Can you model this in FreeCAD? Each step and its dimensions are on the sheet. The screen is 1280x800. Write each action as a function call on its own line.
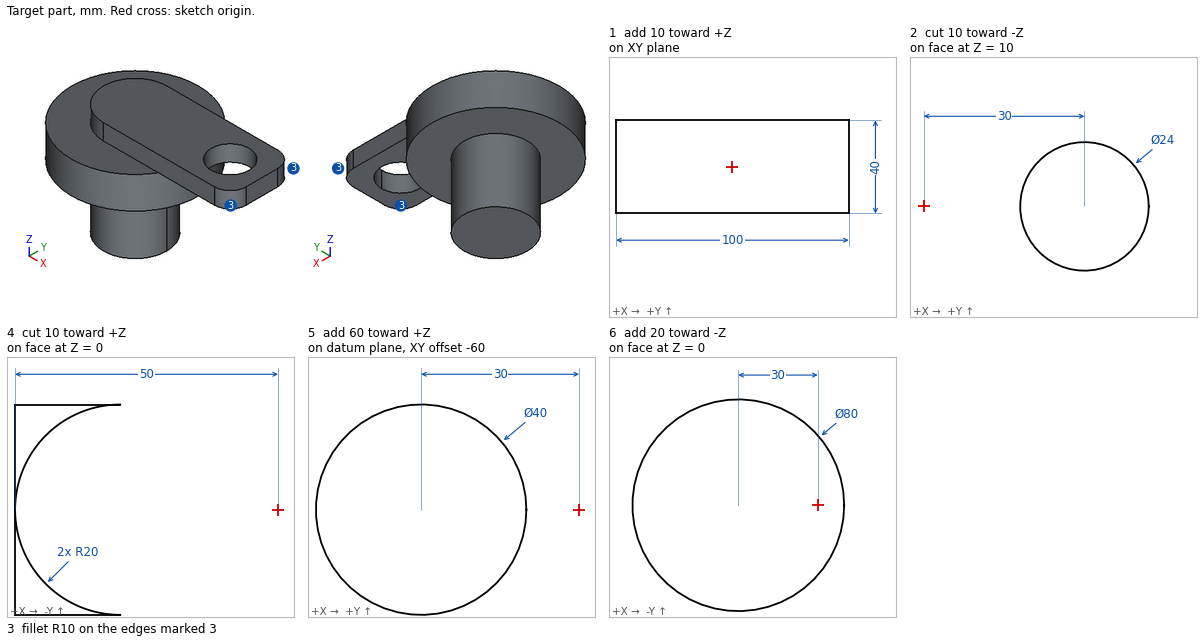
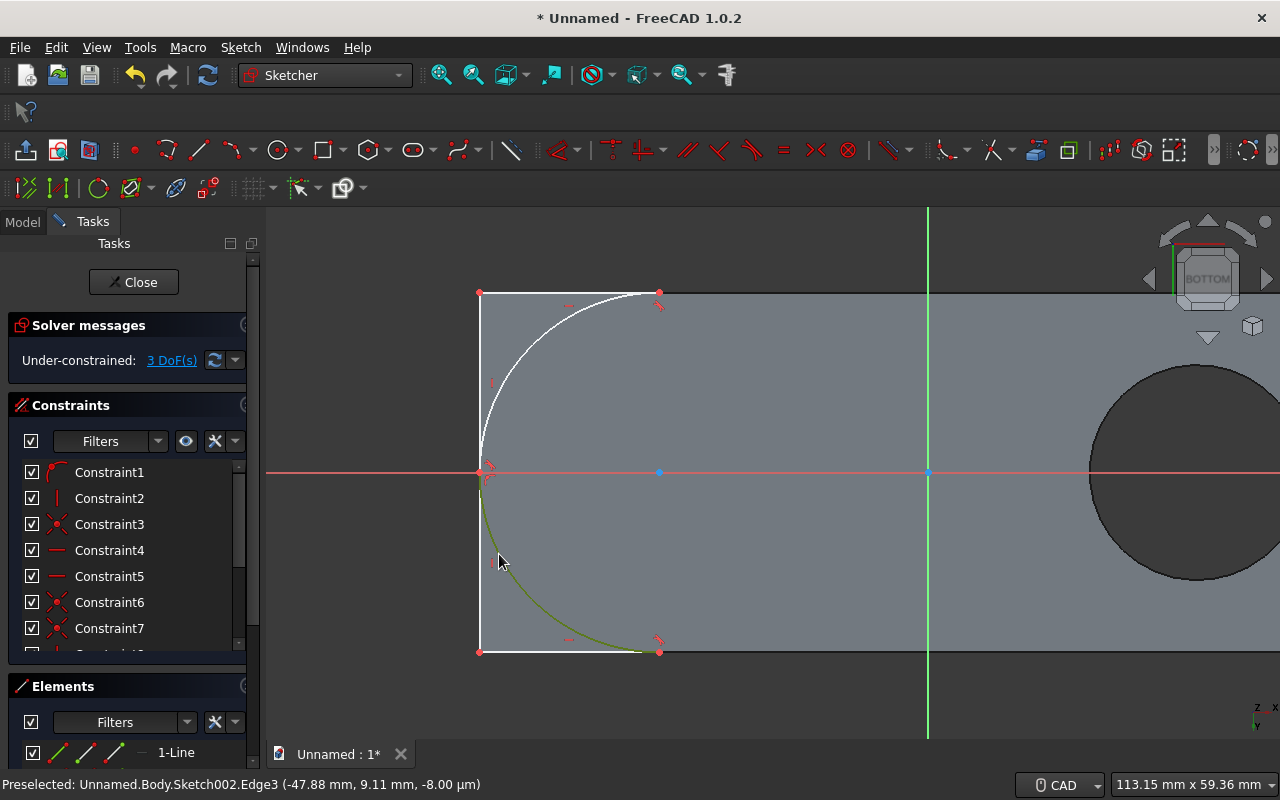
click(578, 312)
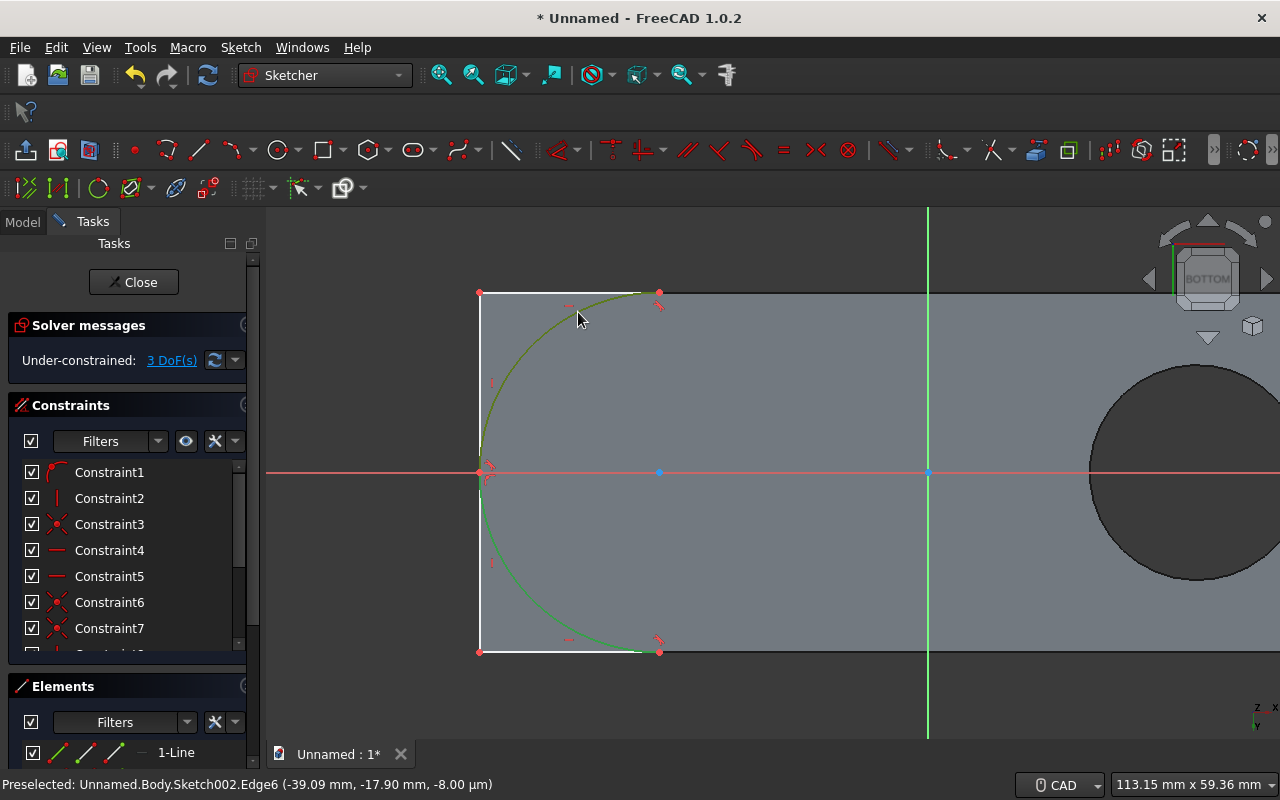
click(784, 150)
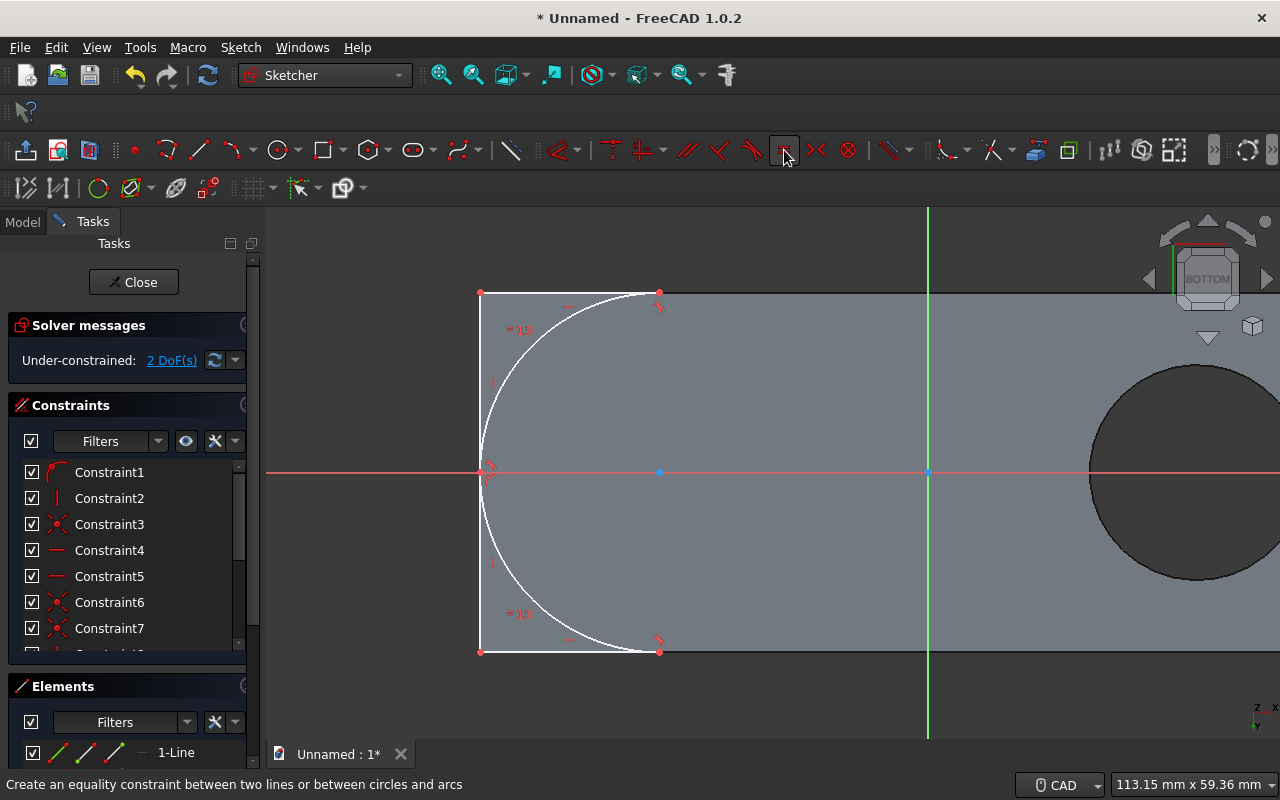
click(500, 554)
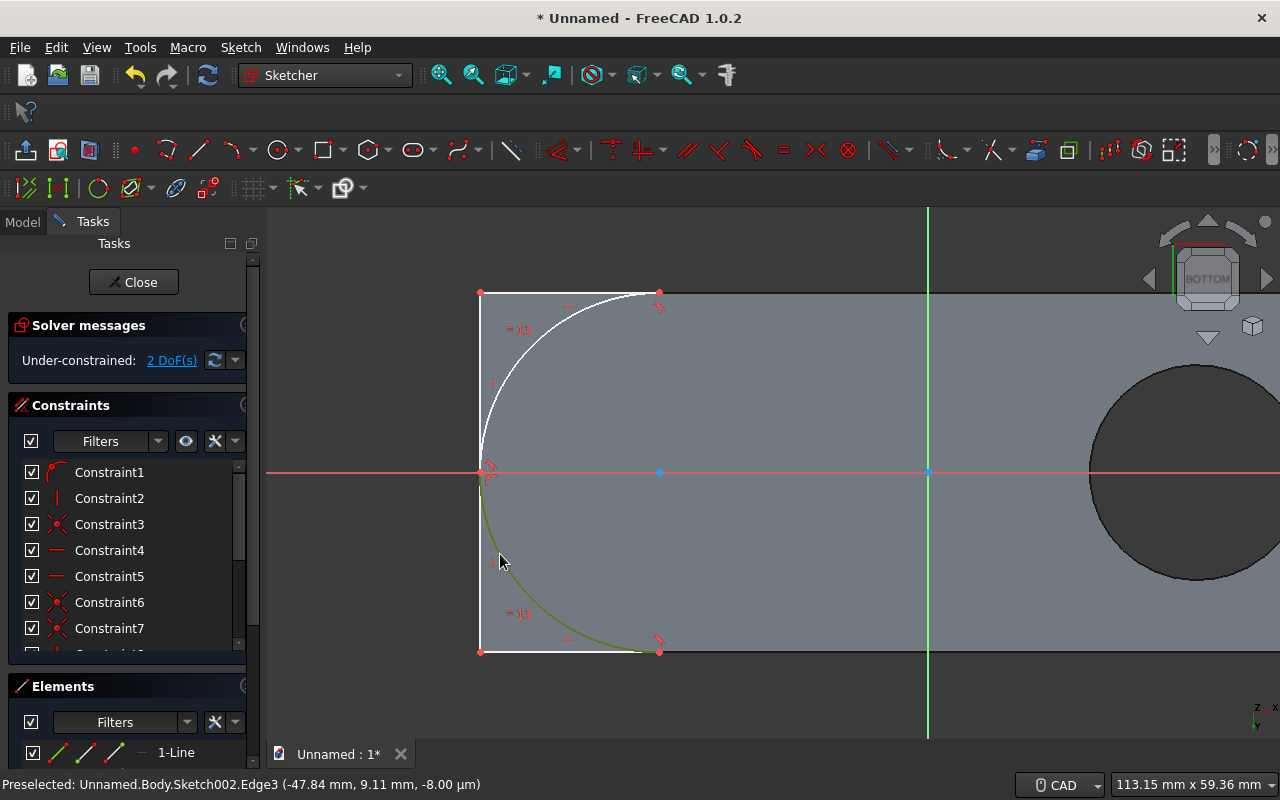
click(580, 150)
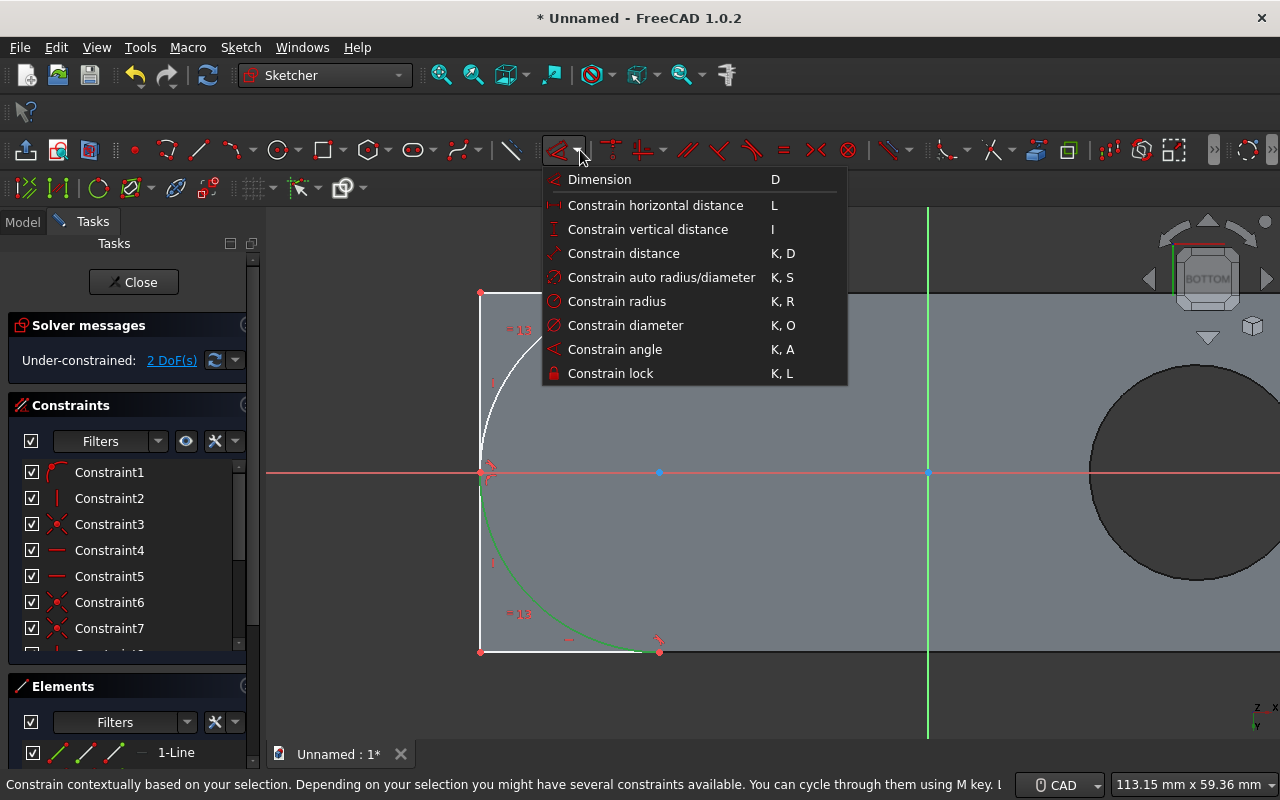
click(695, 301)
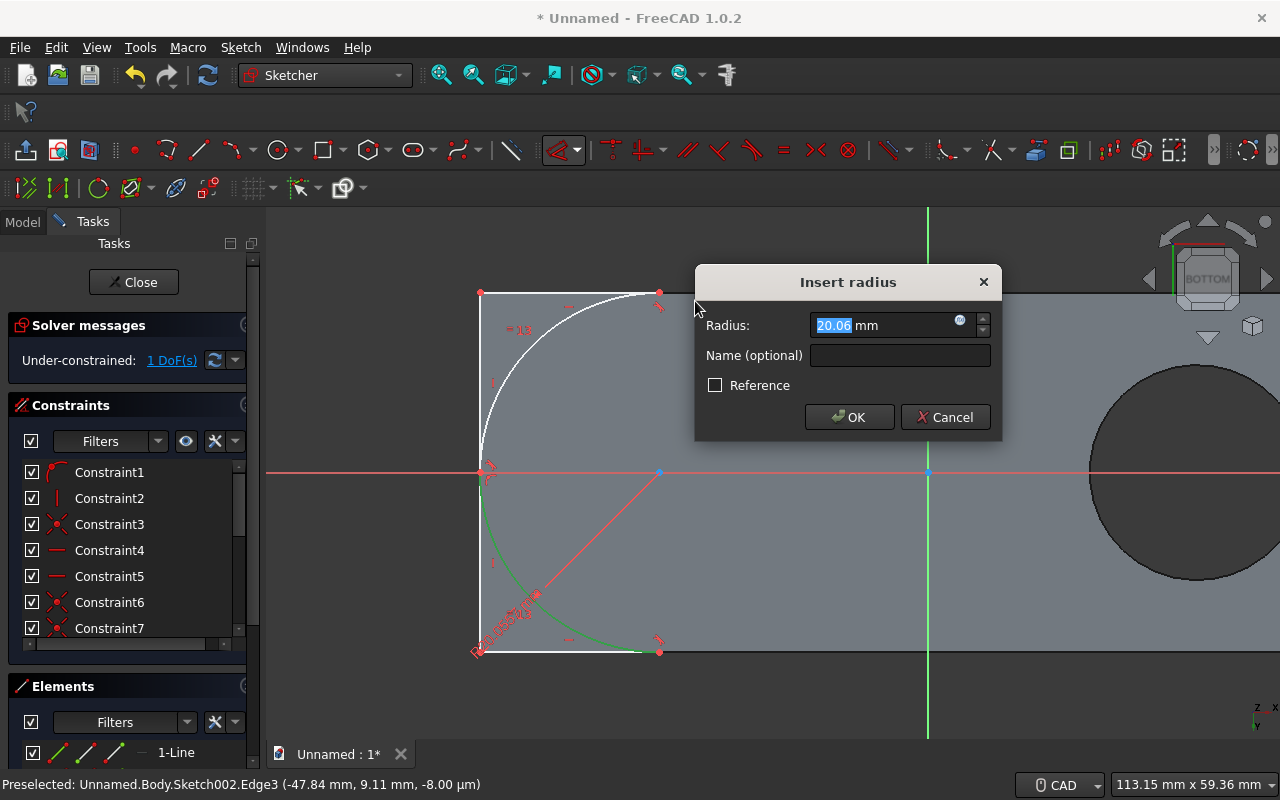
text(20)
key(Return)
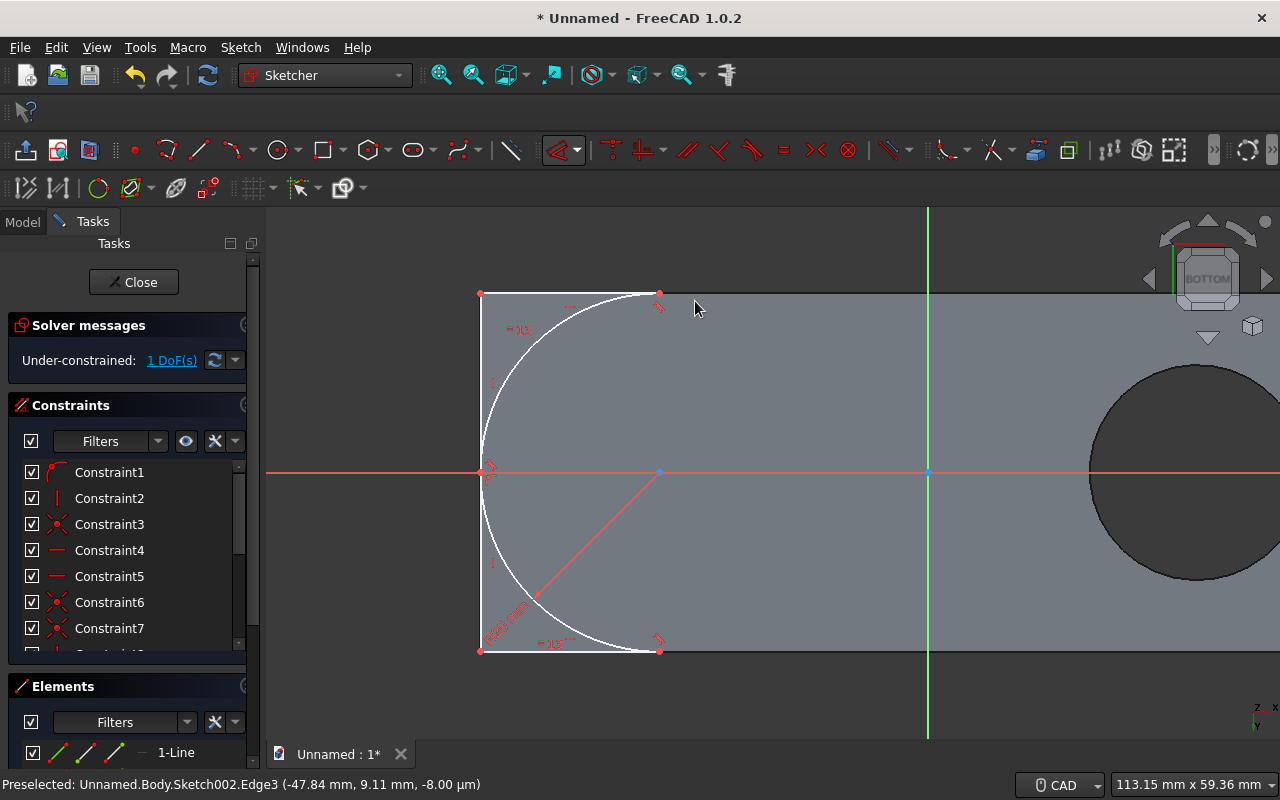
click(481, 473)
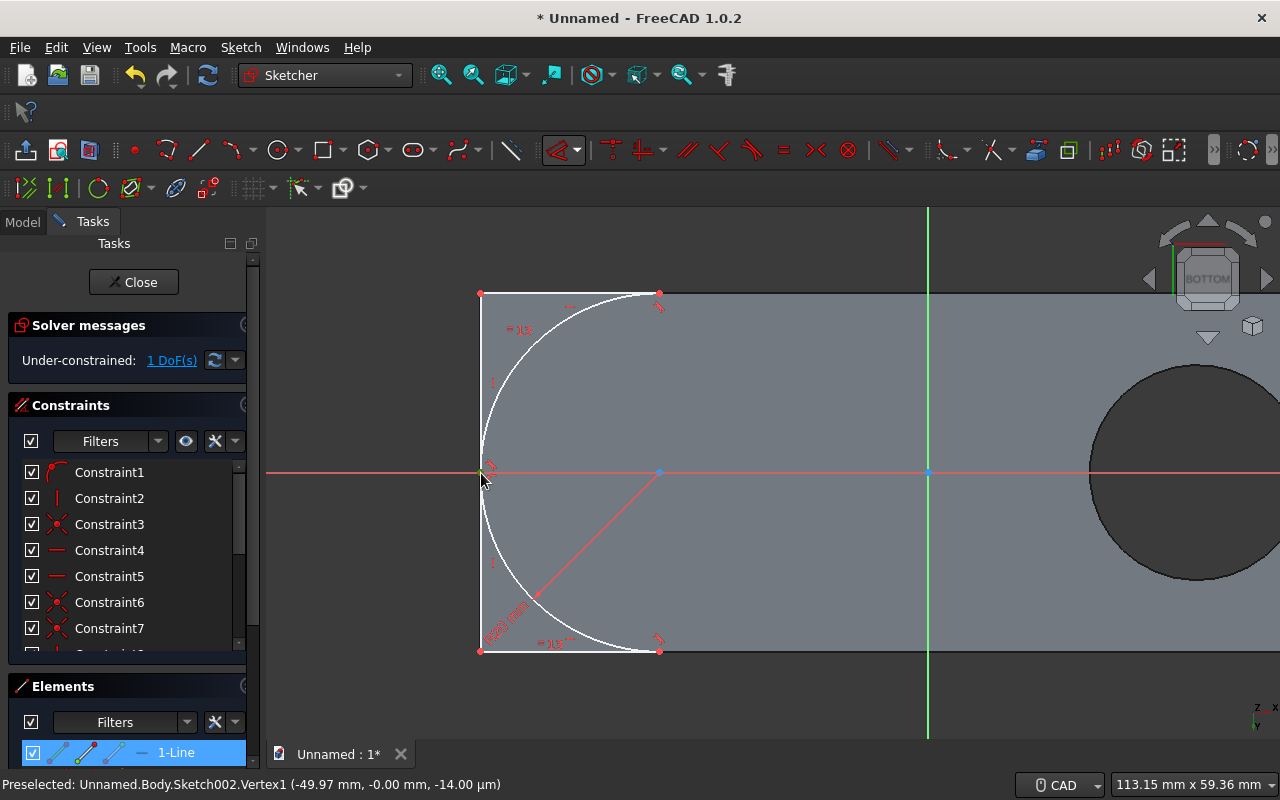
click(580, 150)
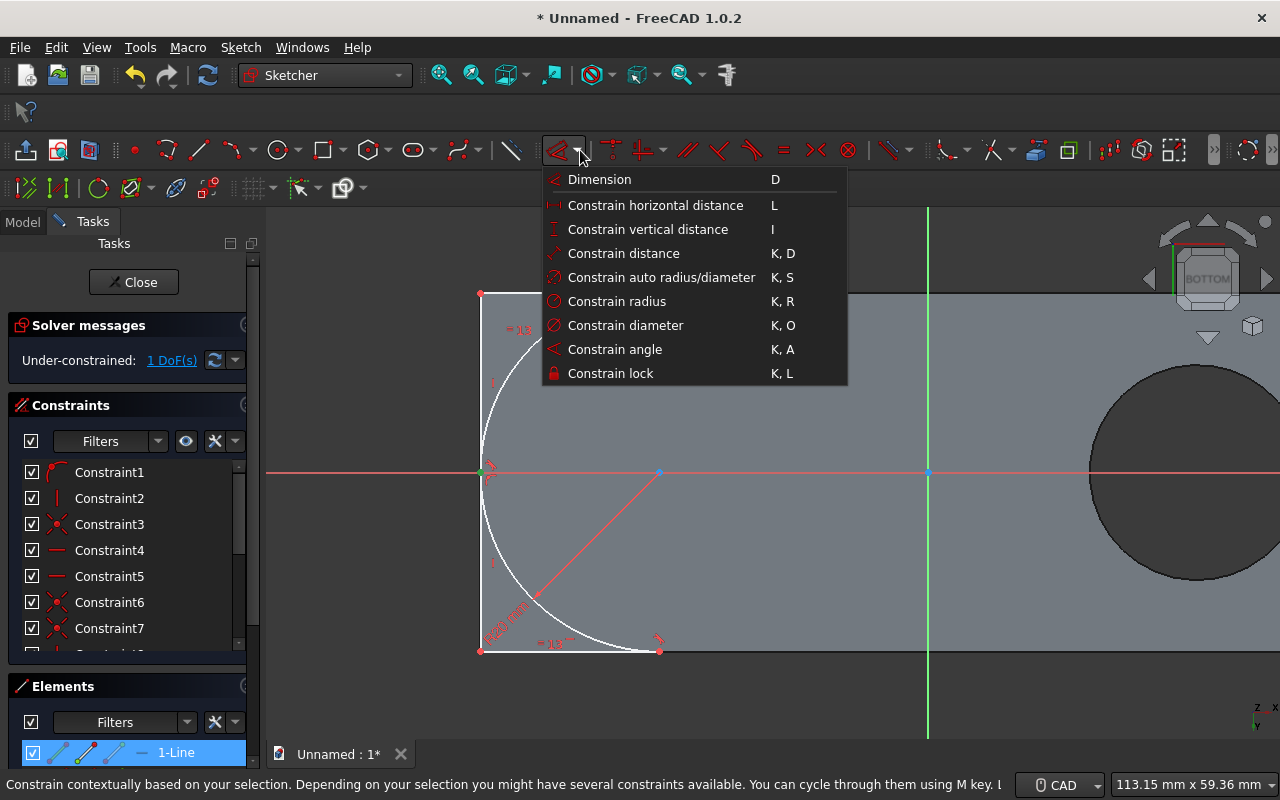
click(695, 205)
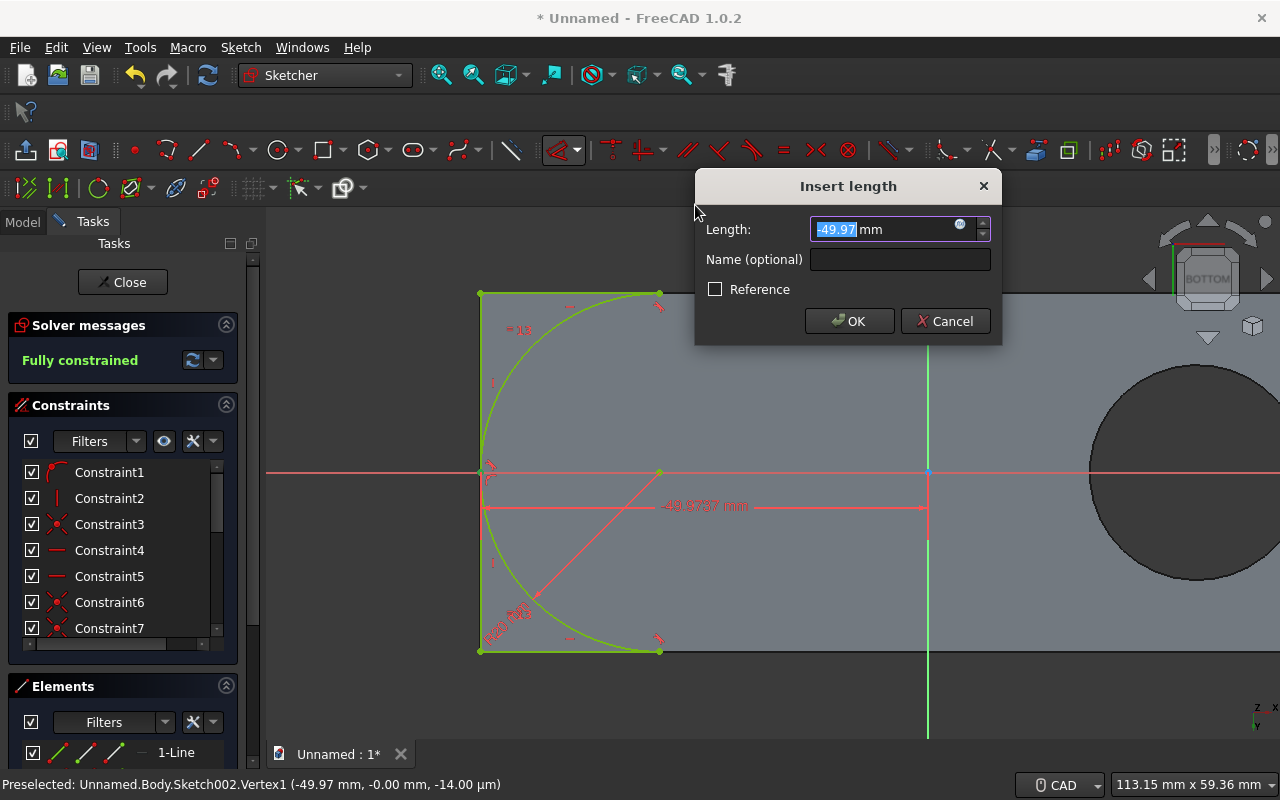
text(-50)
key(Return)